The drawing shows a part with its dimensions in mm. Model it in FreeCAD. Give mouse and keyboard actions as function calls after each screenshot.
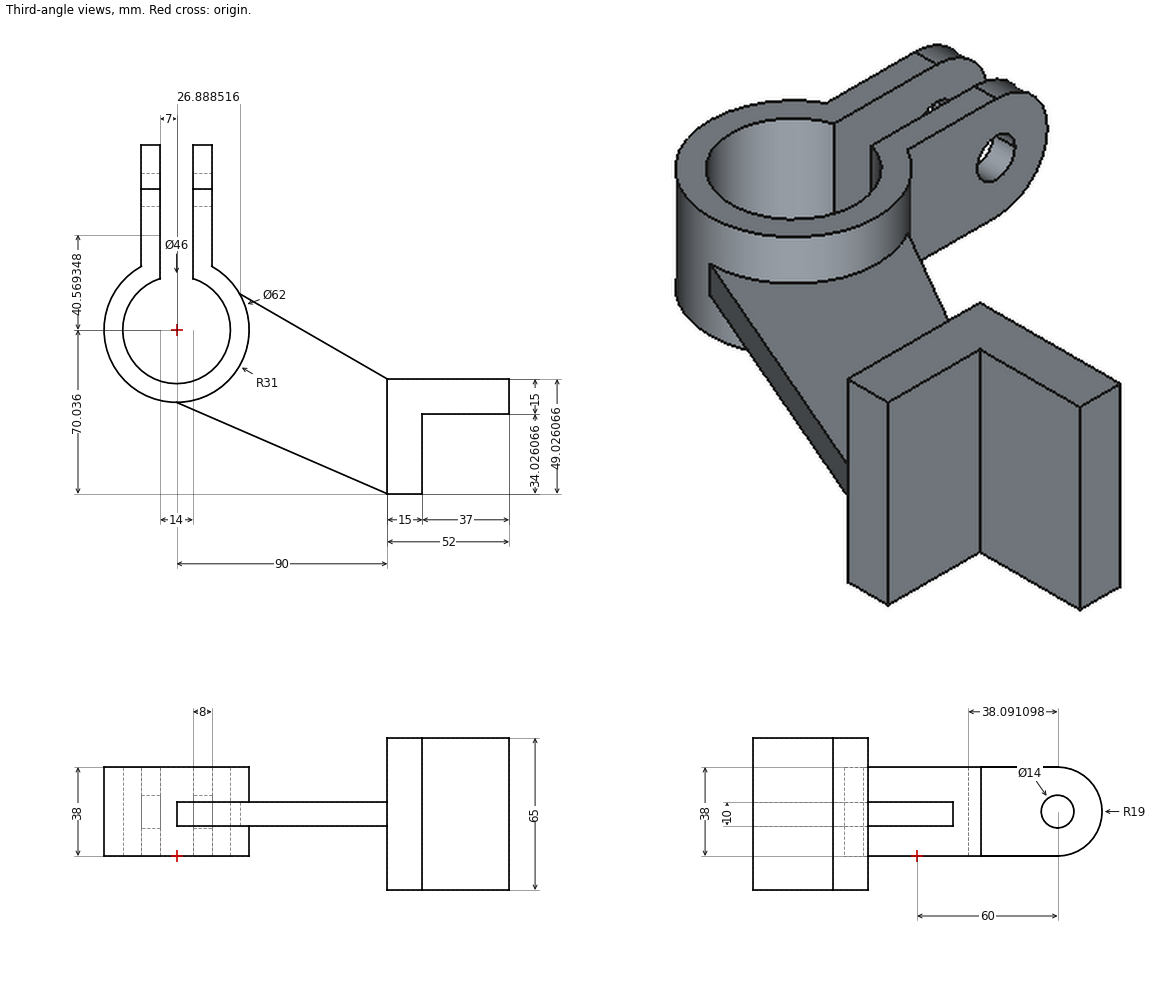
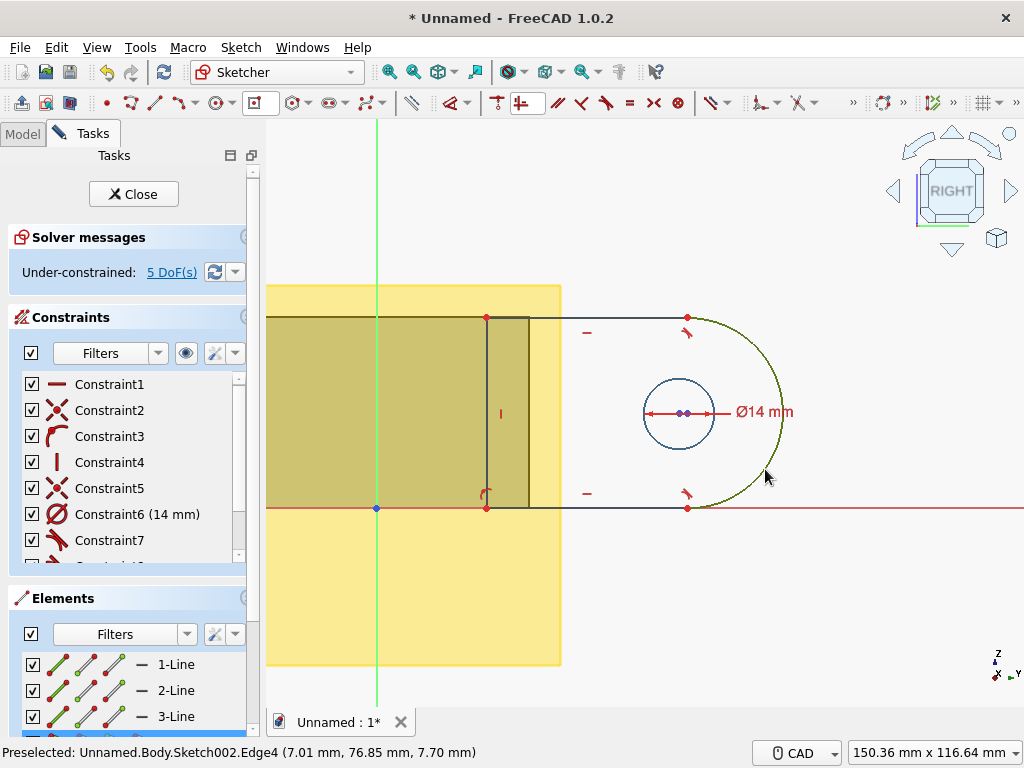
key(c)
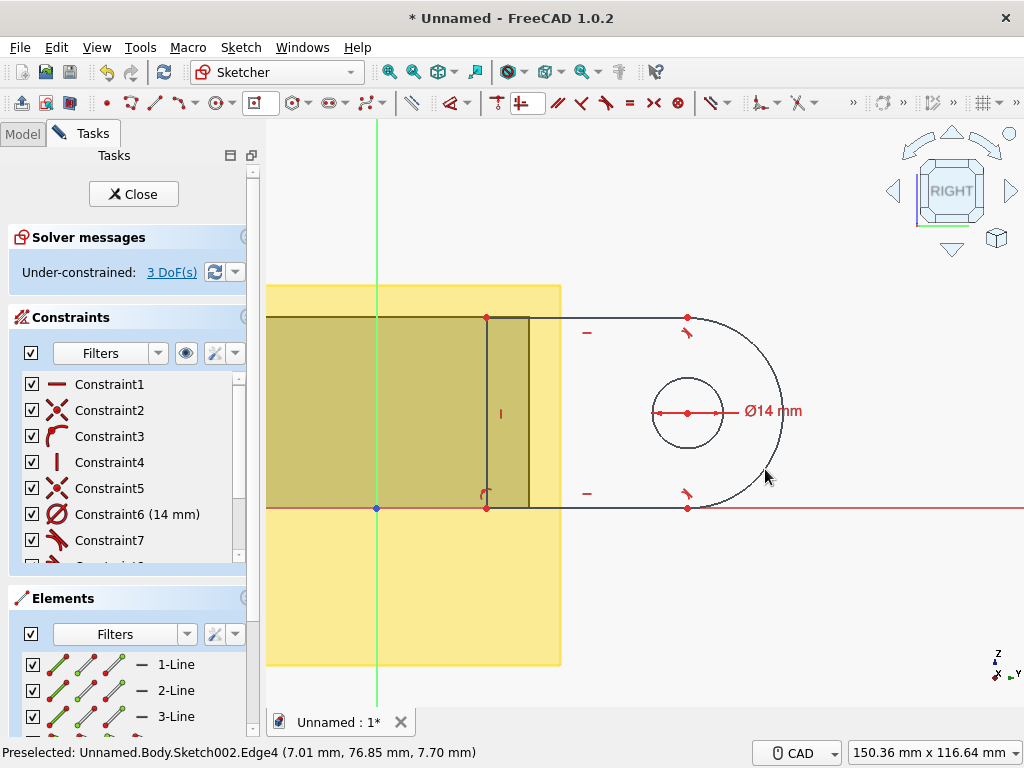
click(450, 104)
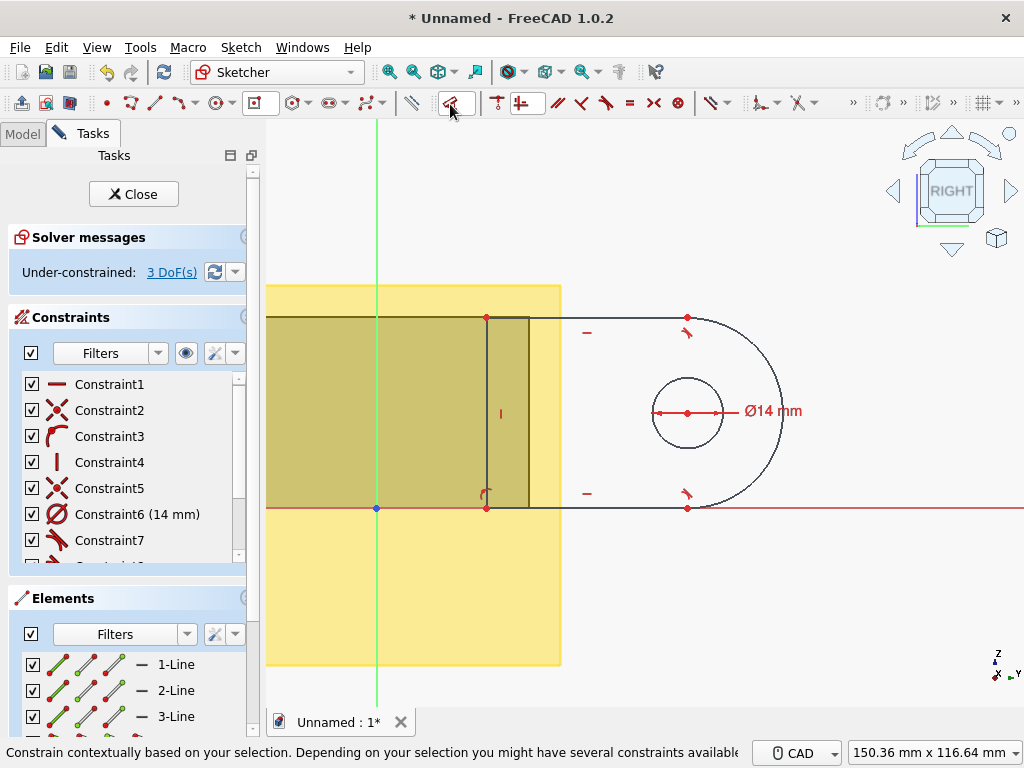
click(765, 469)
click(791, 488)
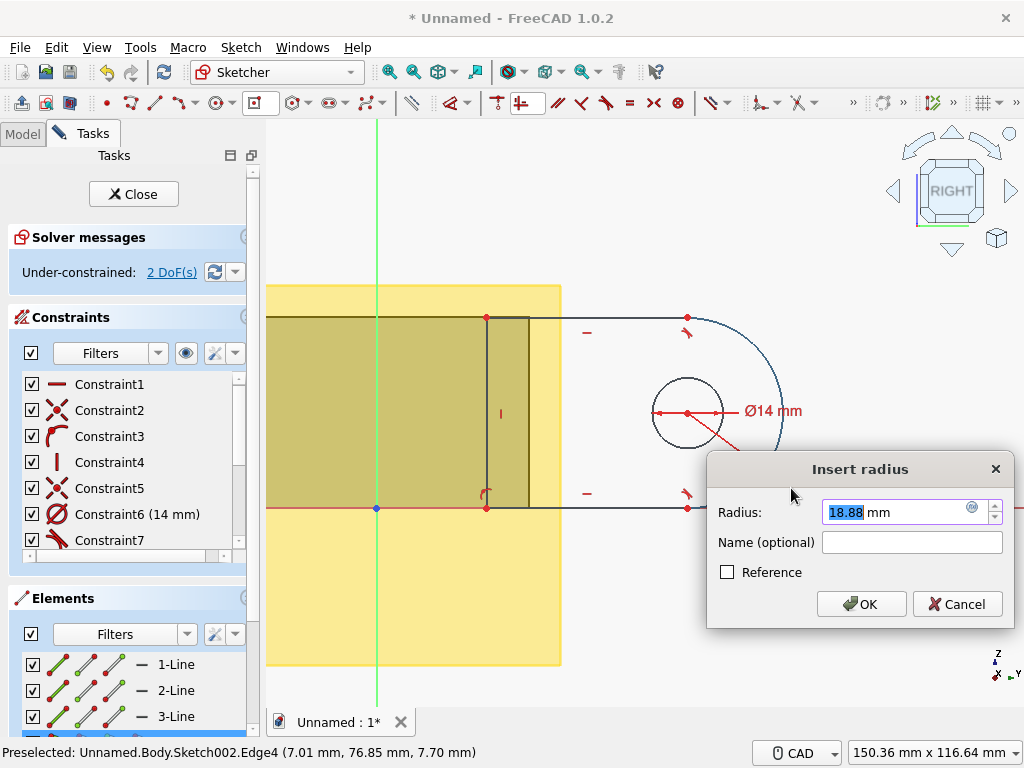
text(19)
key(Return)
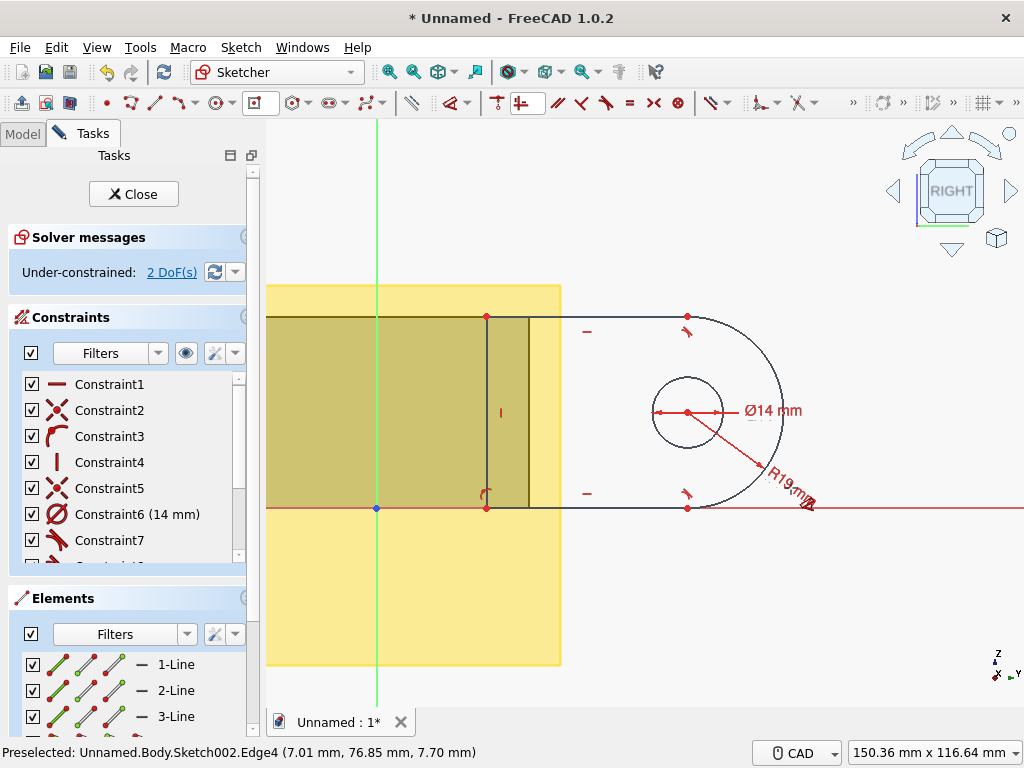
click(688, 413)
click(532, 542)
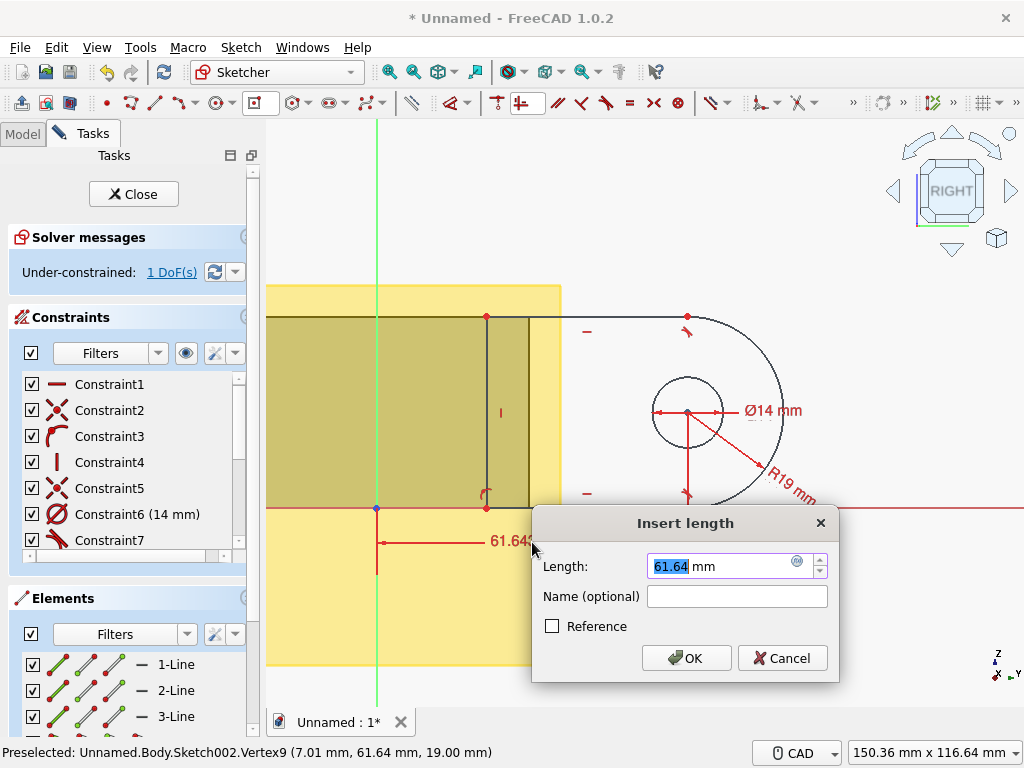
text(60)
key(Return)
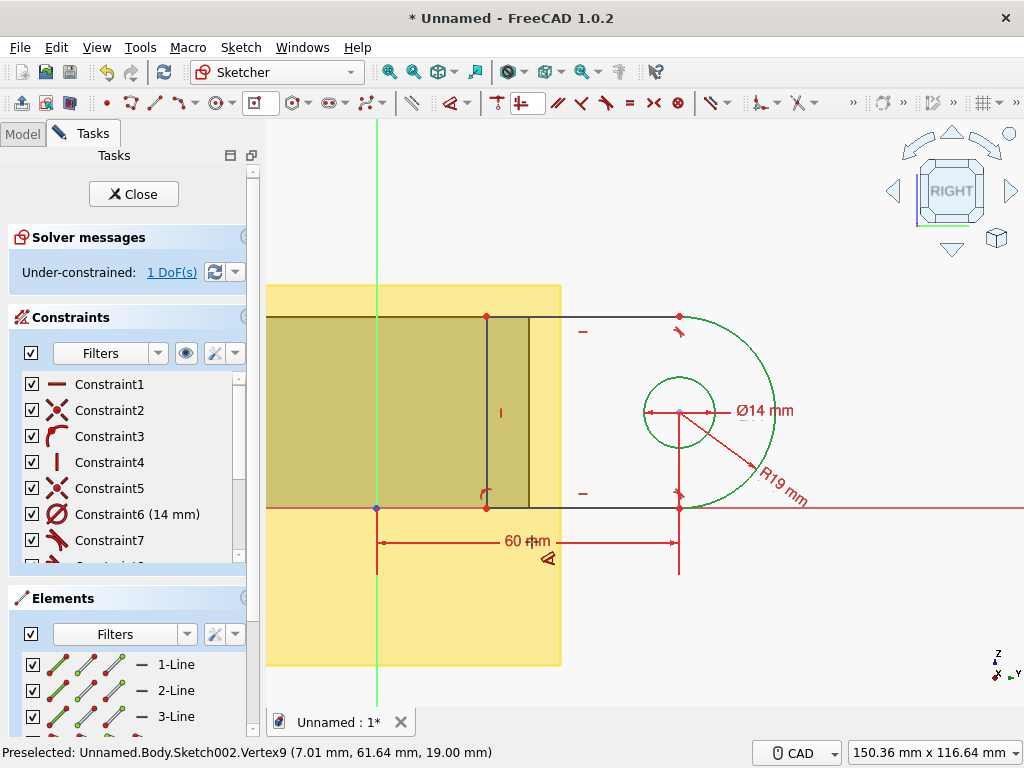
click(622, 317)
click(583, 283)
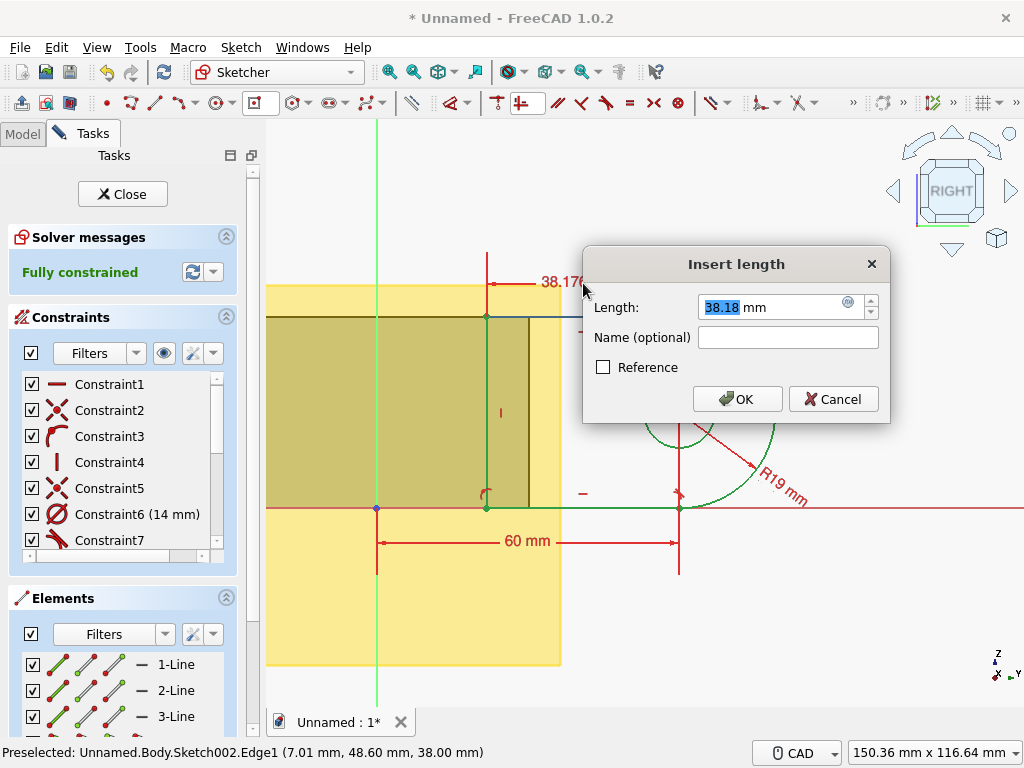
text(38.091098)
key(Return)
key(Escape)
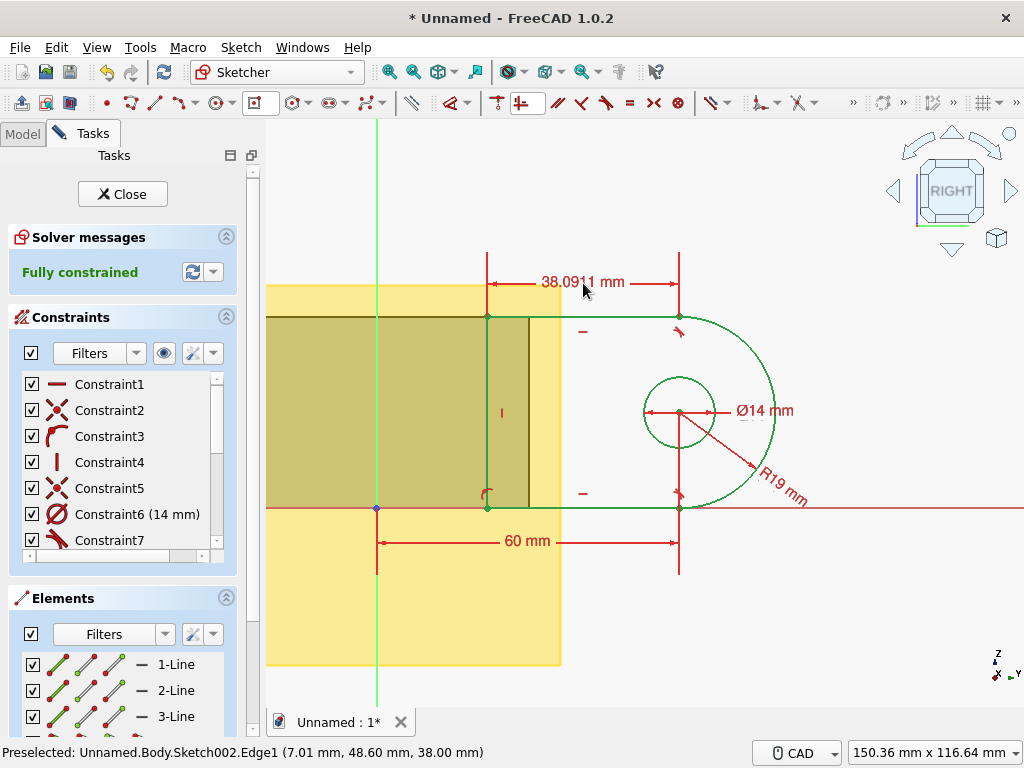
click(123, 194)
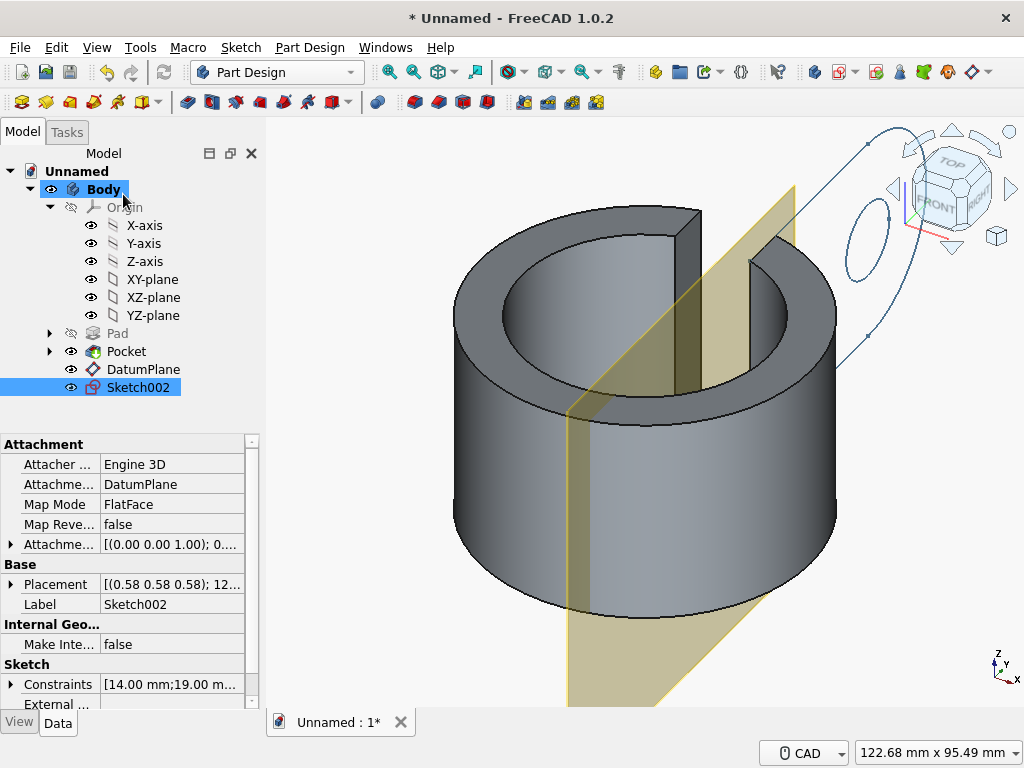
click(22, 102)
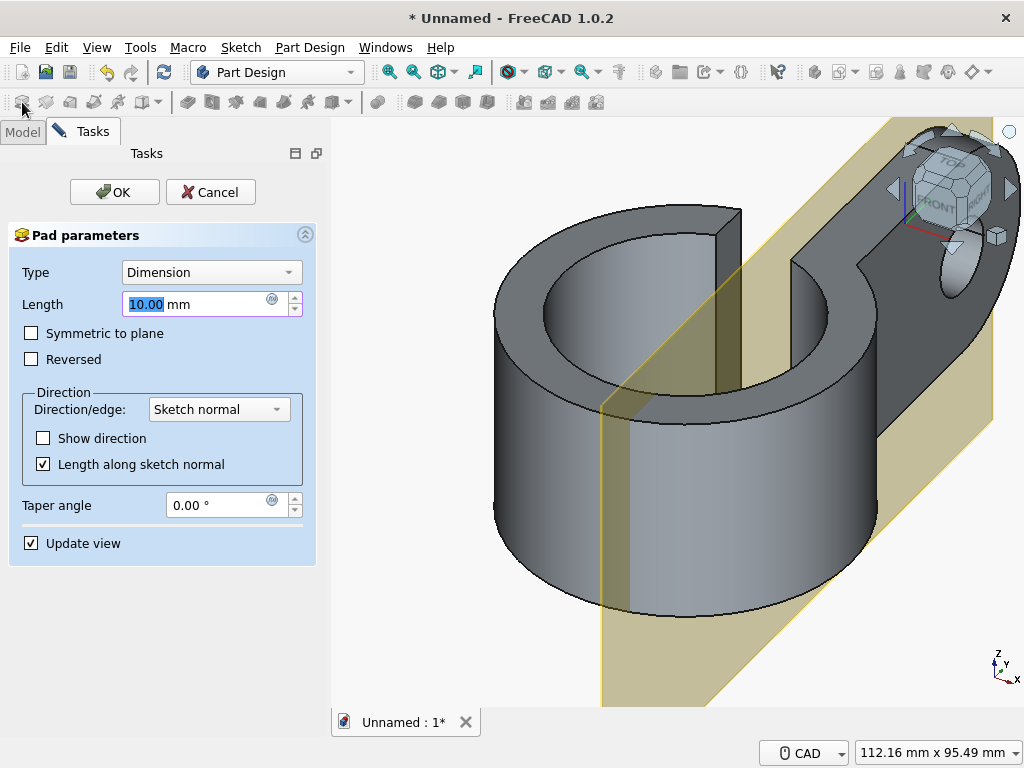
text(8)
key(Tab)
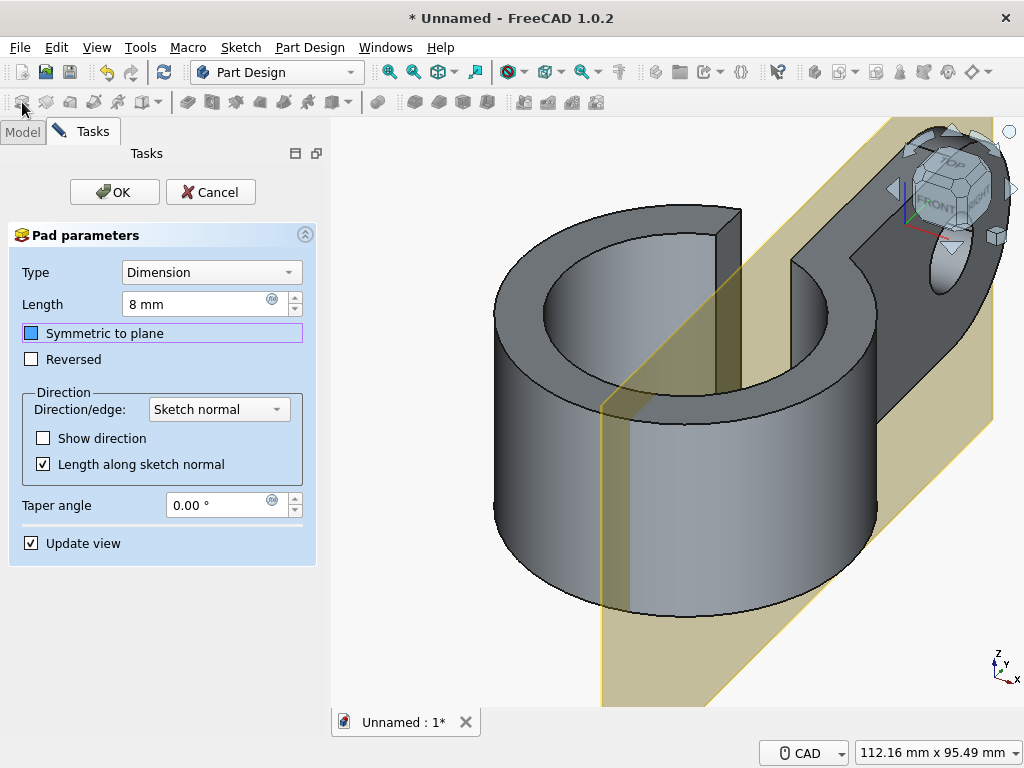
click(115, 192)